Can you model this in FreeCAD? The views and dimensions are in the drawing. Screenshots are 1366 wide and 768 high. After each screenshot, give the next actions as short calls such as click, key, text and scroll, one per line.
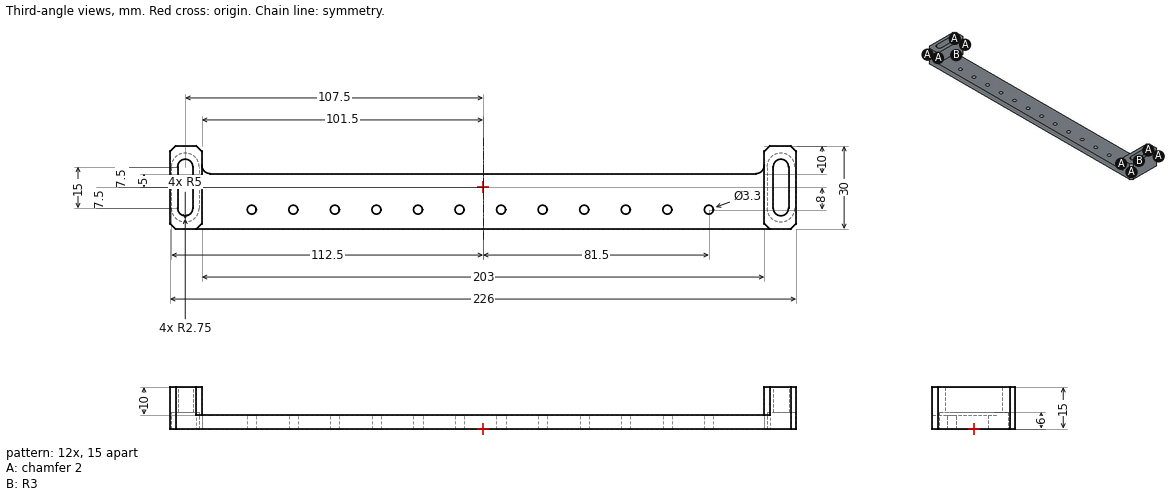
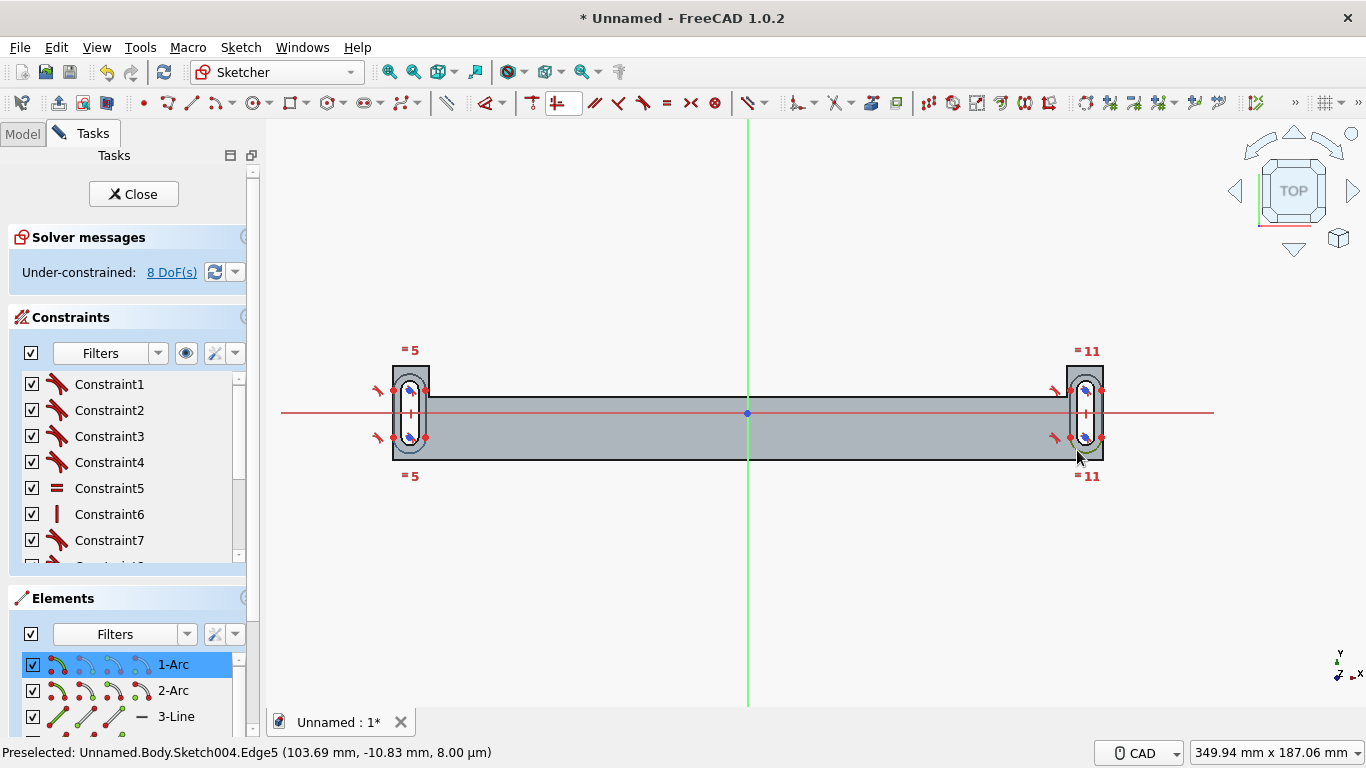
key(e)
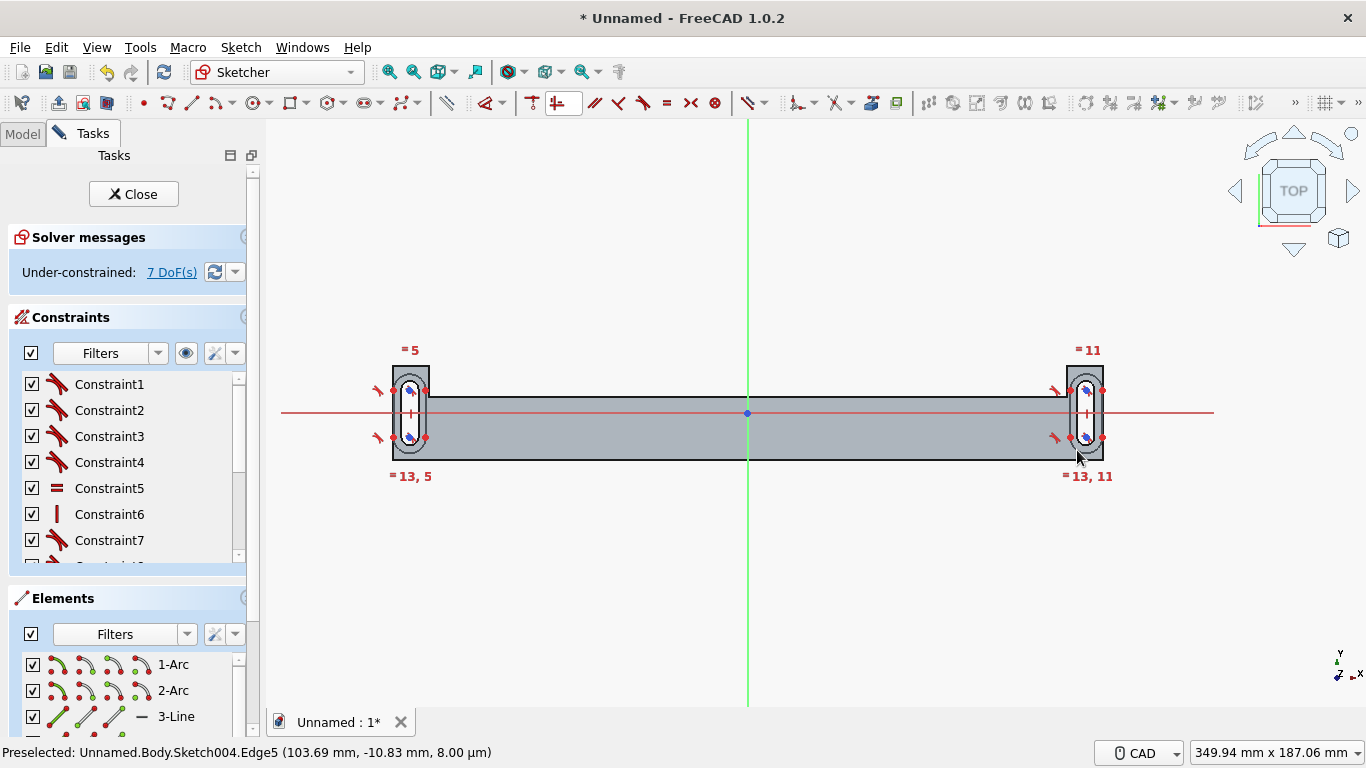
click(410, 437)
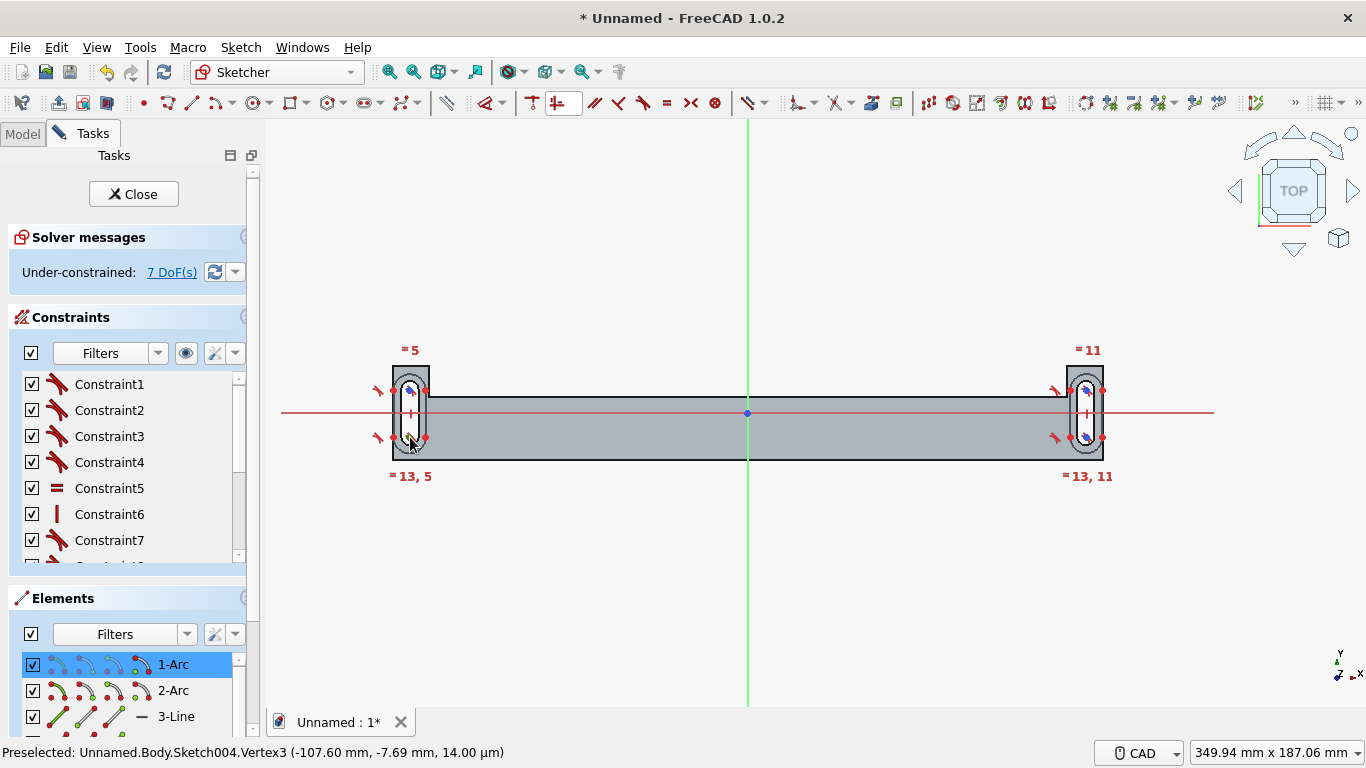
click(1086, 437)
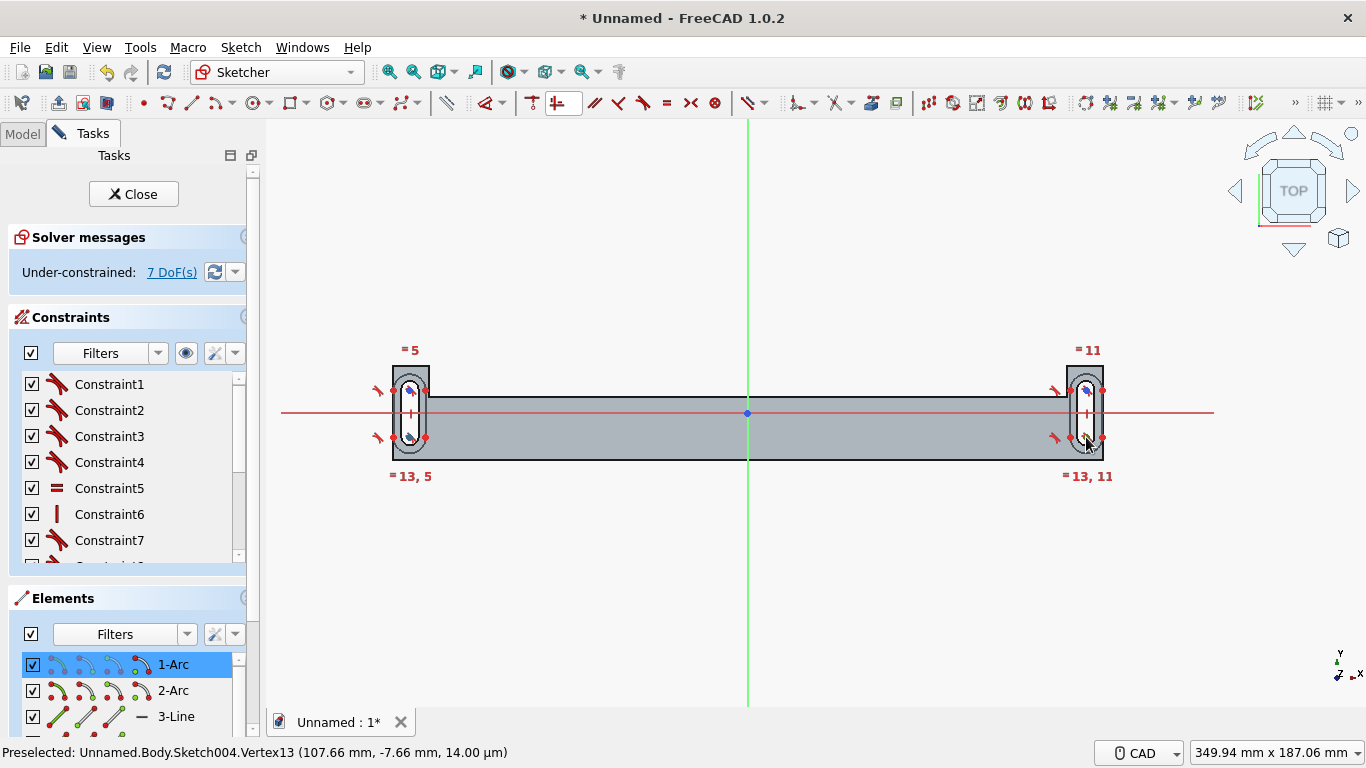
click(748, 641)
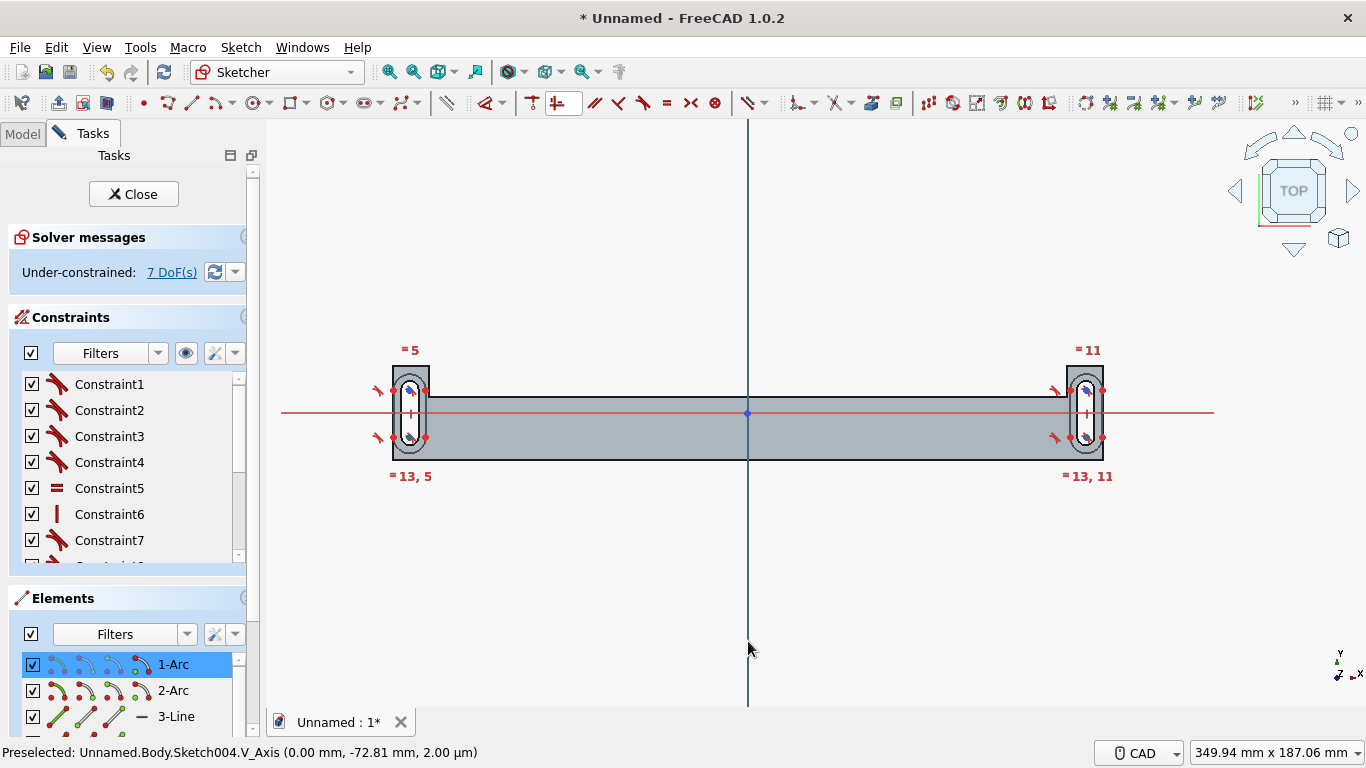
click(692, 104)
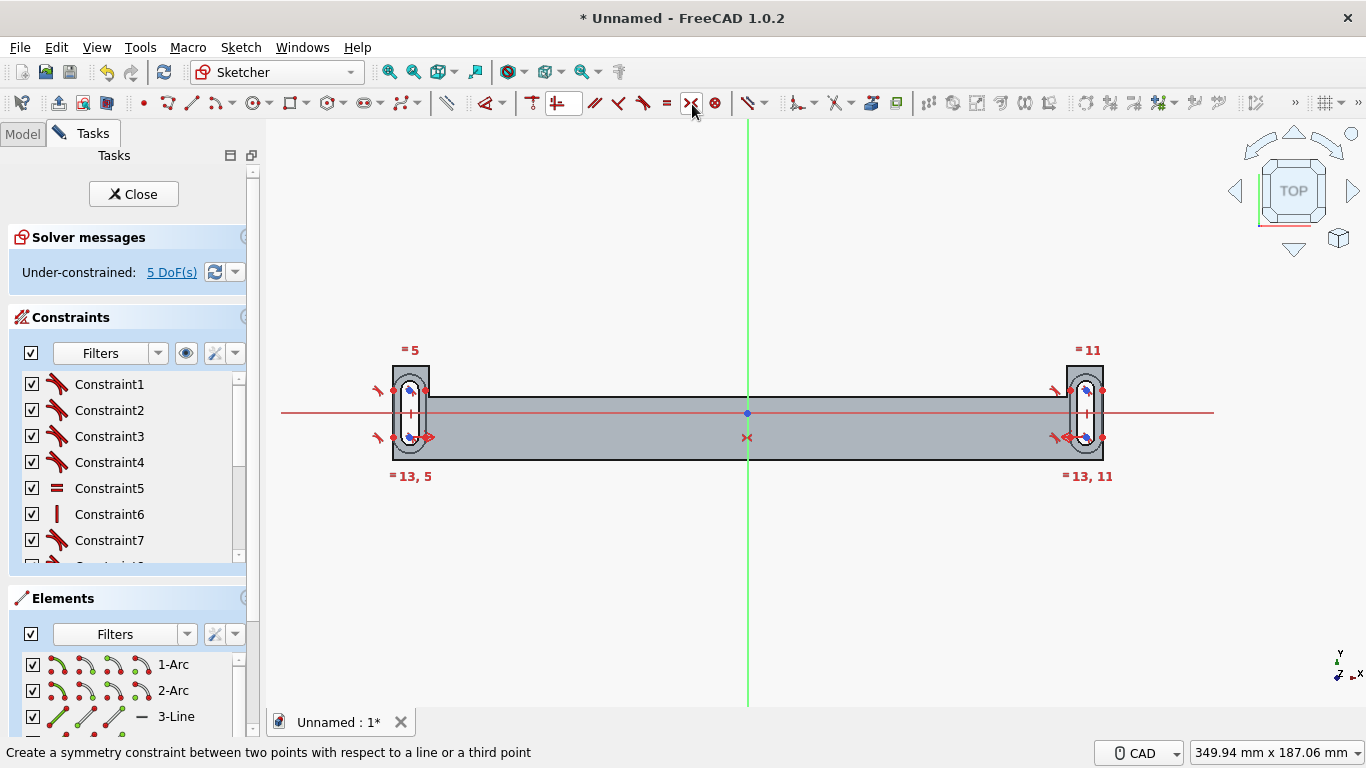
key(d)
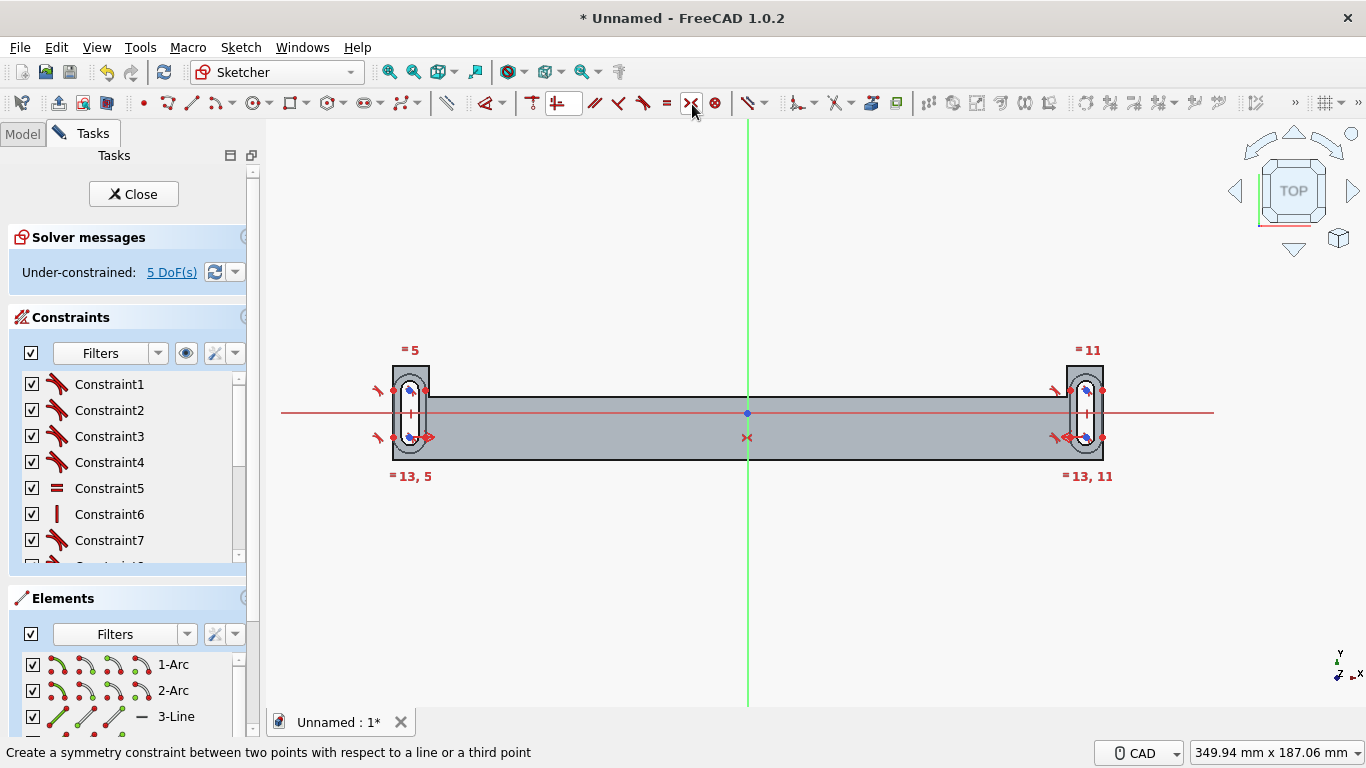
scroll(400, 450, up, 5)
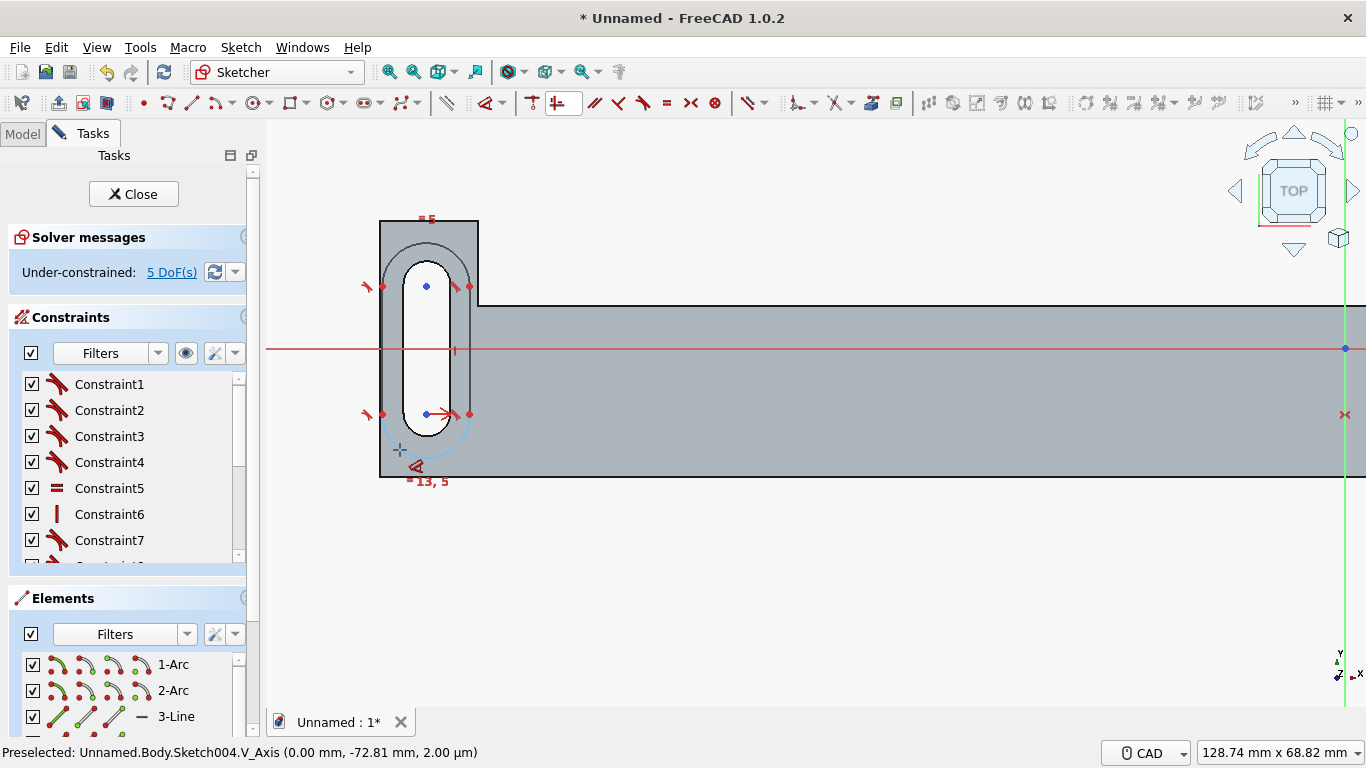
click(400, 450)
click(381, 476)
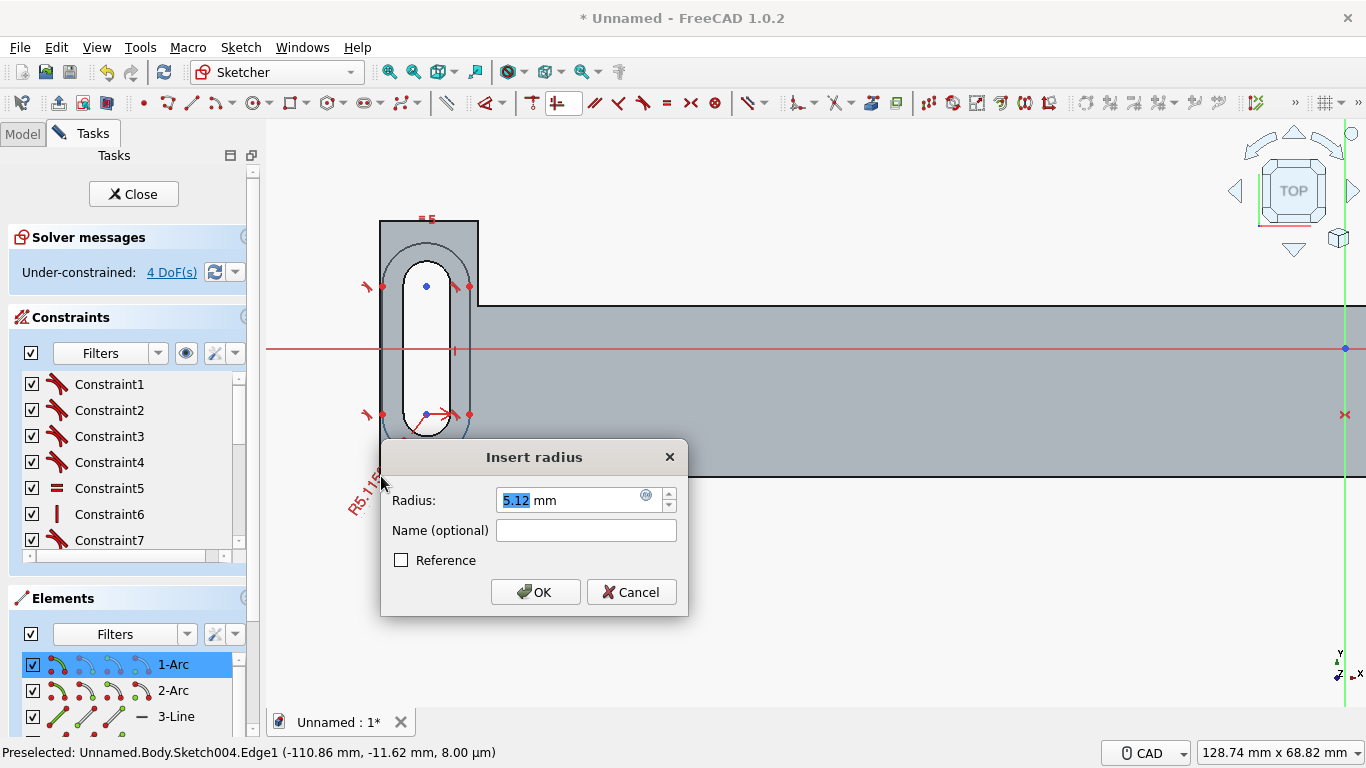
text(5)
key(Return)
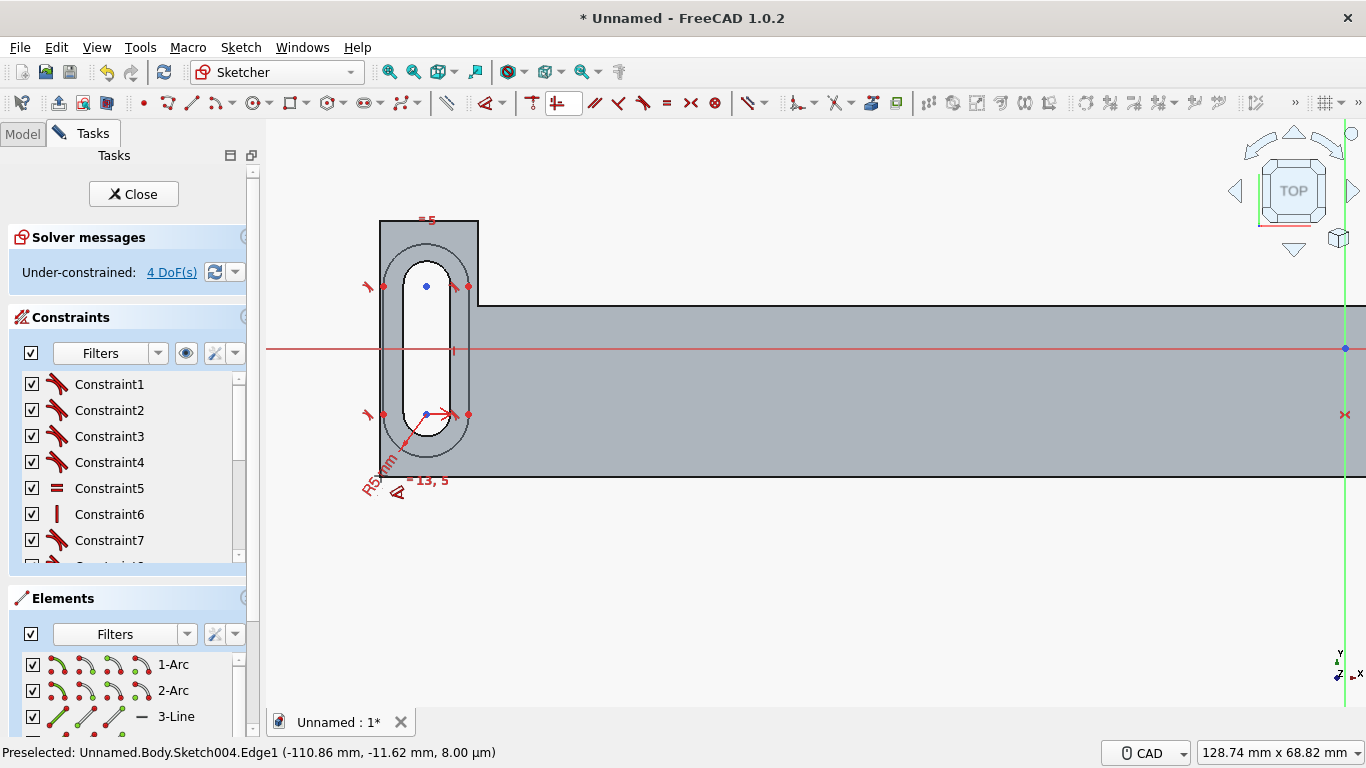
click(383, 376)
click(349, 321)